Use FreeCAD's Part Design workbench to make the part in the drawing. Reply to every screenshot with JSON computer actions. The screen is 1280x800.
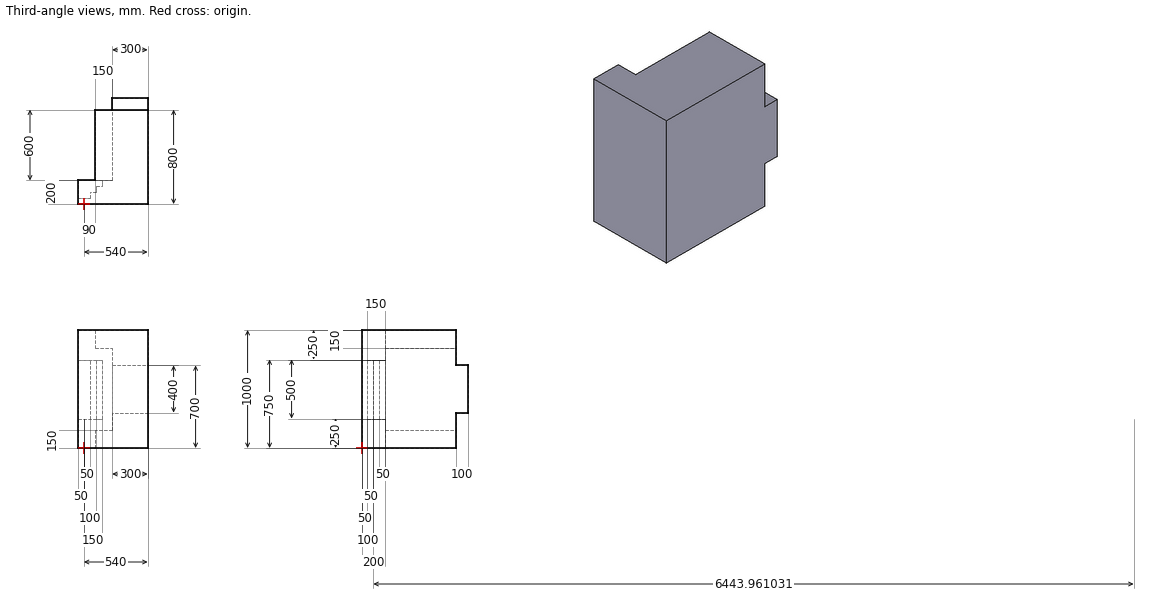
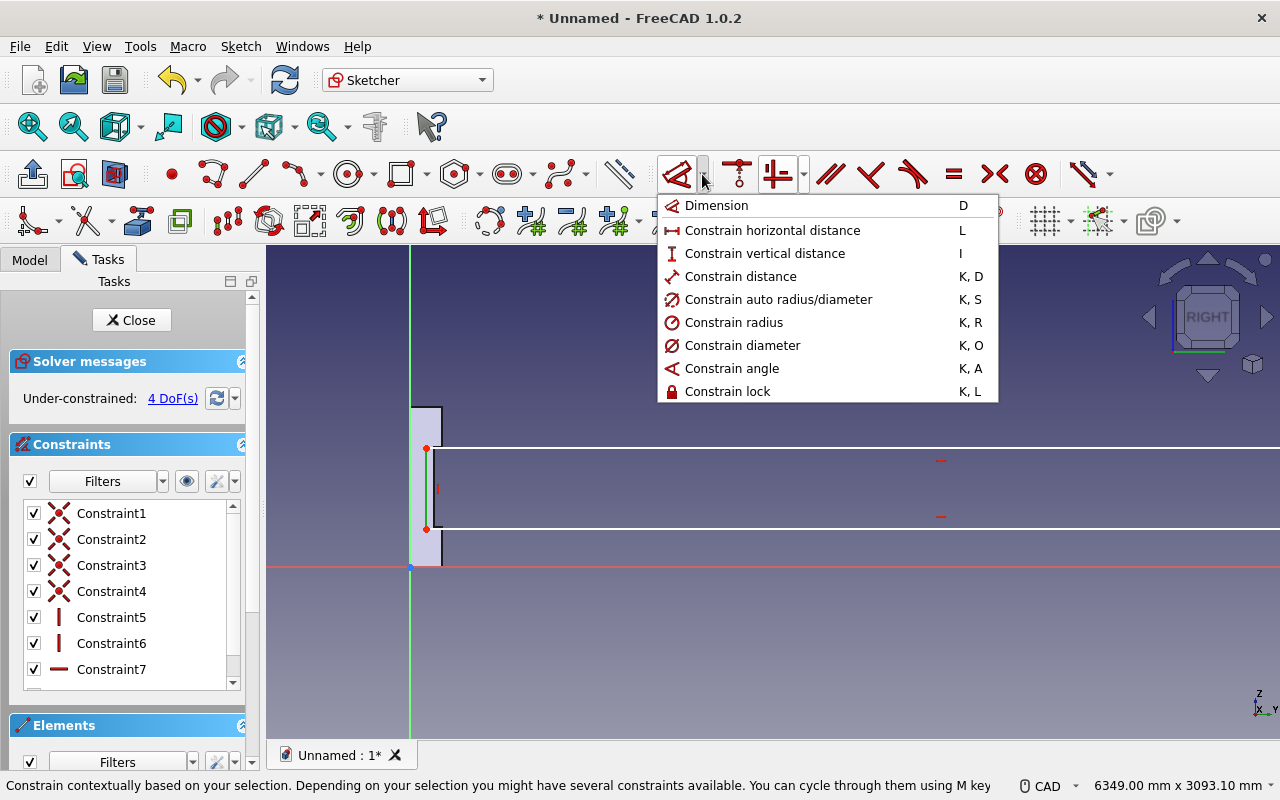
{"action": "left_click", "coordinate": [828, 254]}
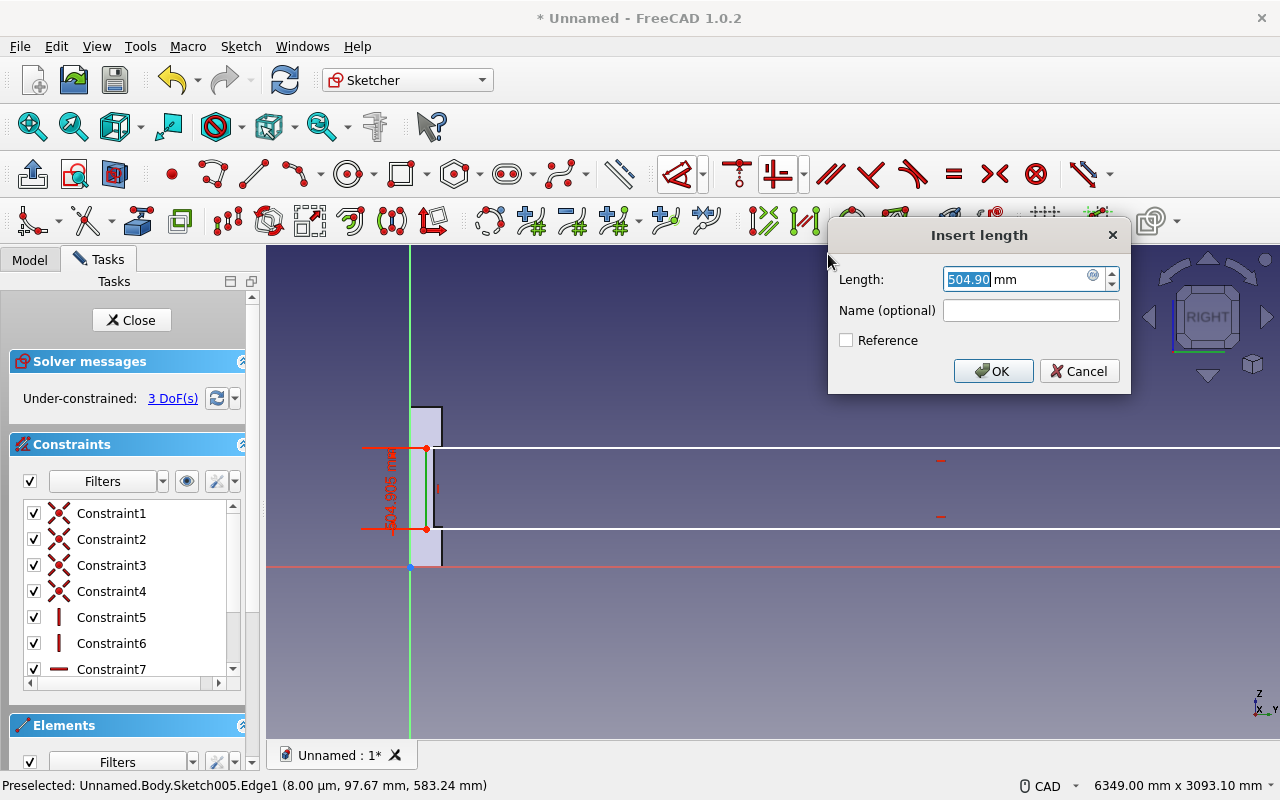
{"action": "type", "text": "500"}
{"action": "key", "text": "Return"}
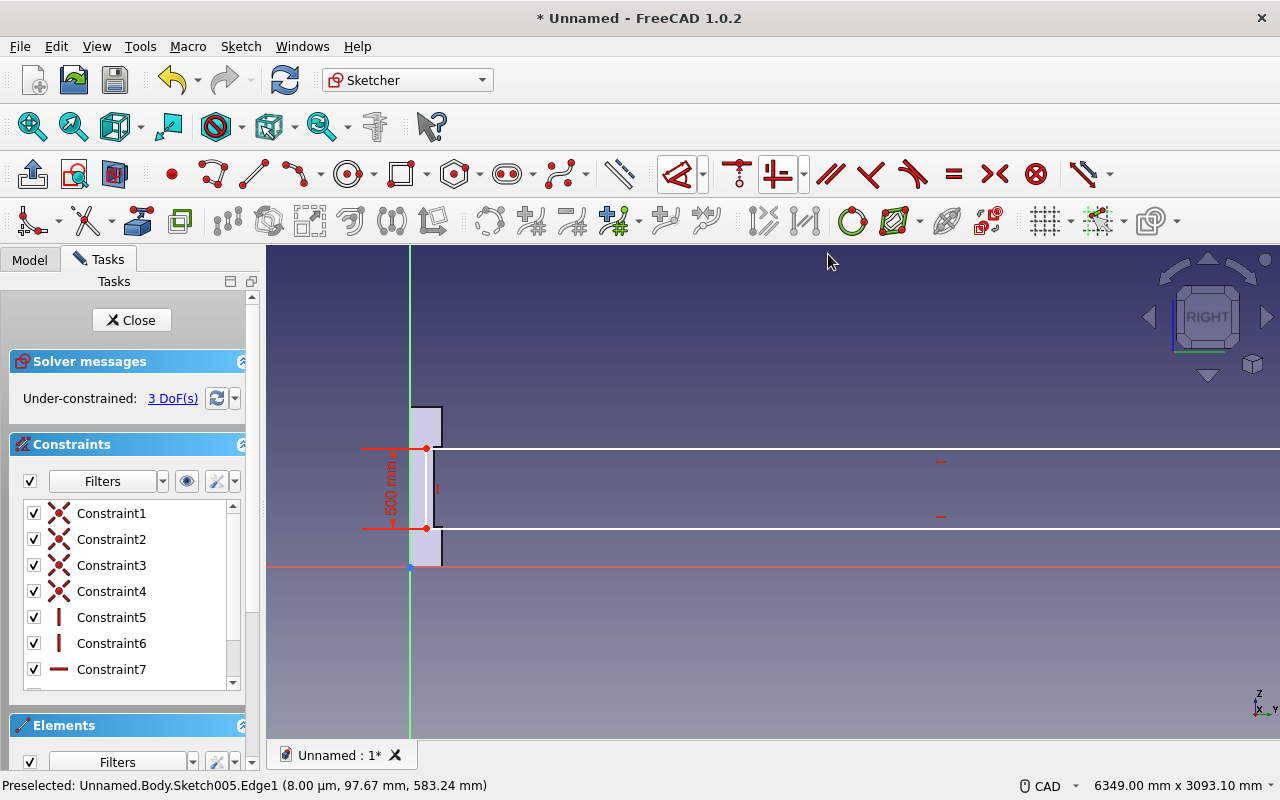
{"action": "scroll", "coordinate": [426, 449], "scroll_direction": "up", "scroll_amount": 5}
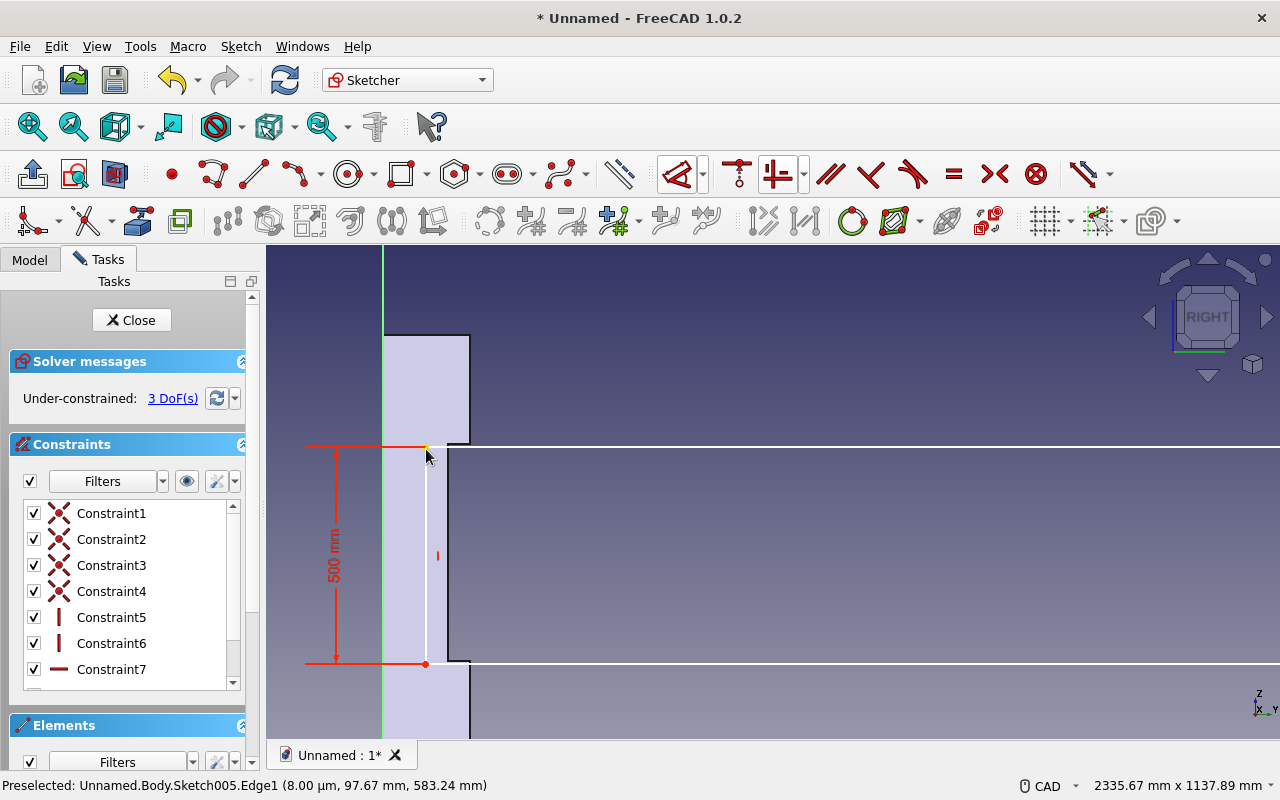
{"action": "left_click", "coordinate": [426, 447]}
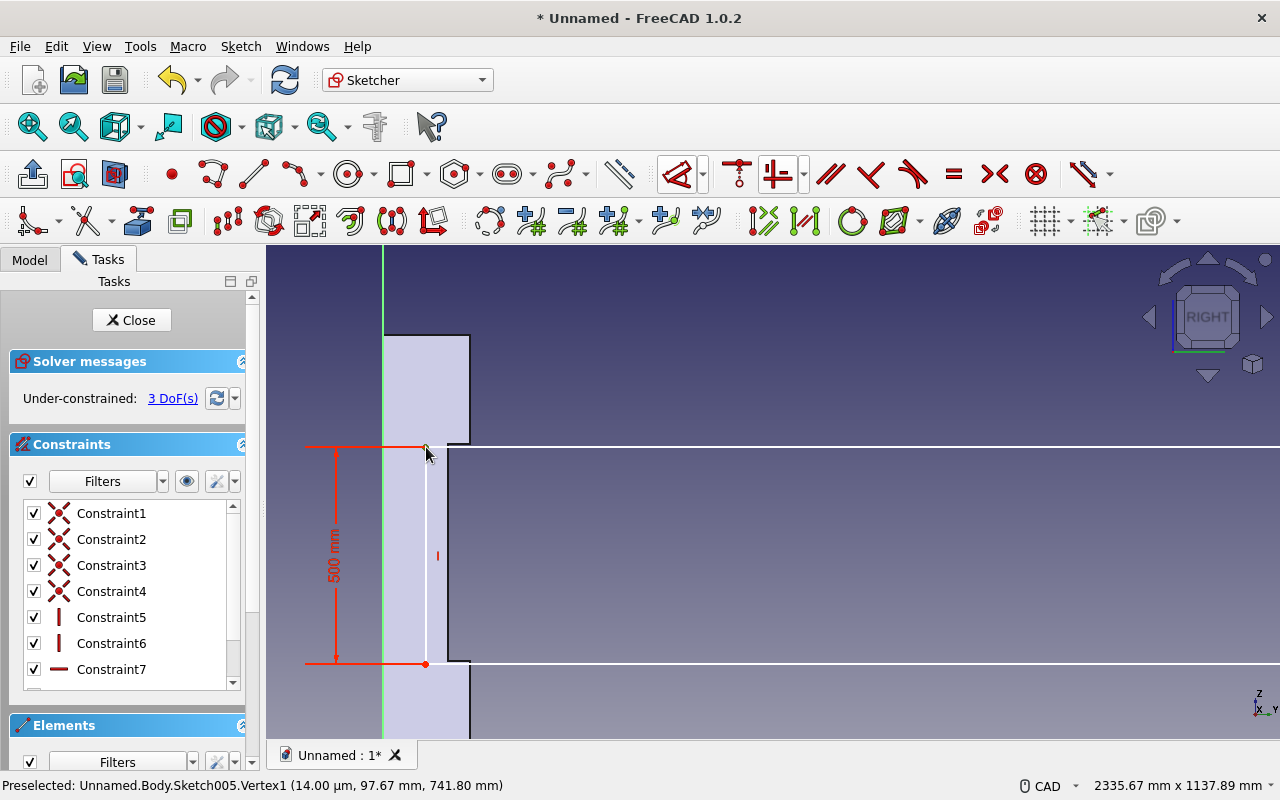
{"action": "left_click", "coordinate": [702, 174]}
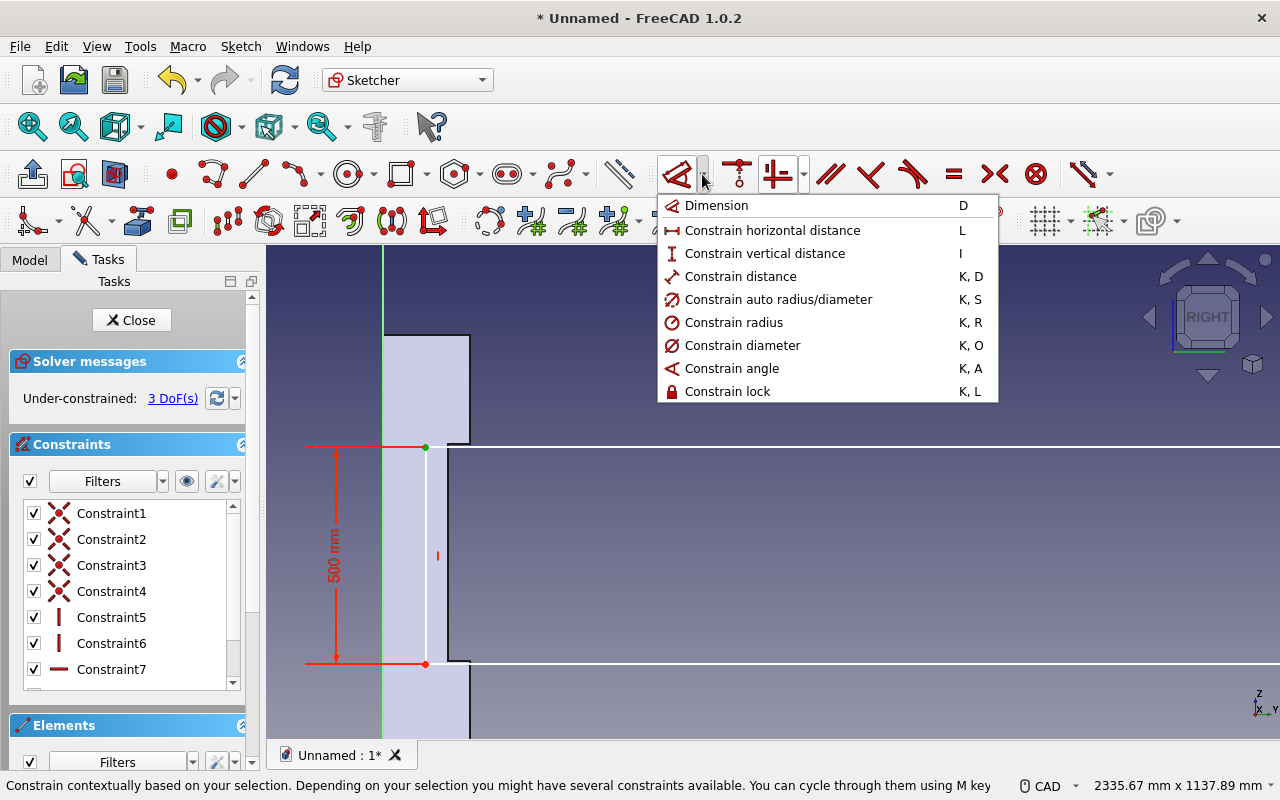
{"action": "left_click", "coordinate": [828, 230]}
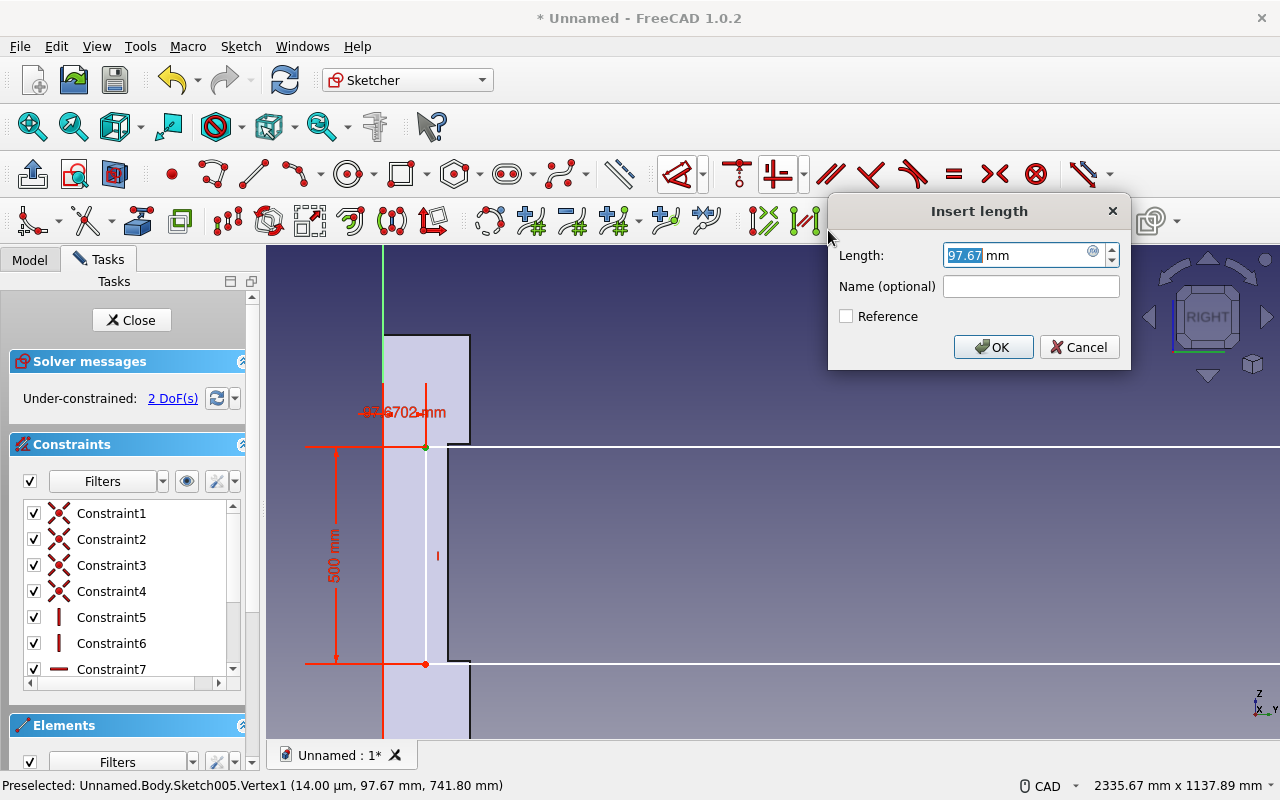
{"action": "type", "text": "100"}
{"action": "key", "text": "Return"}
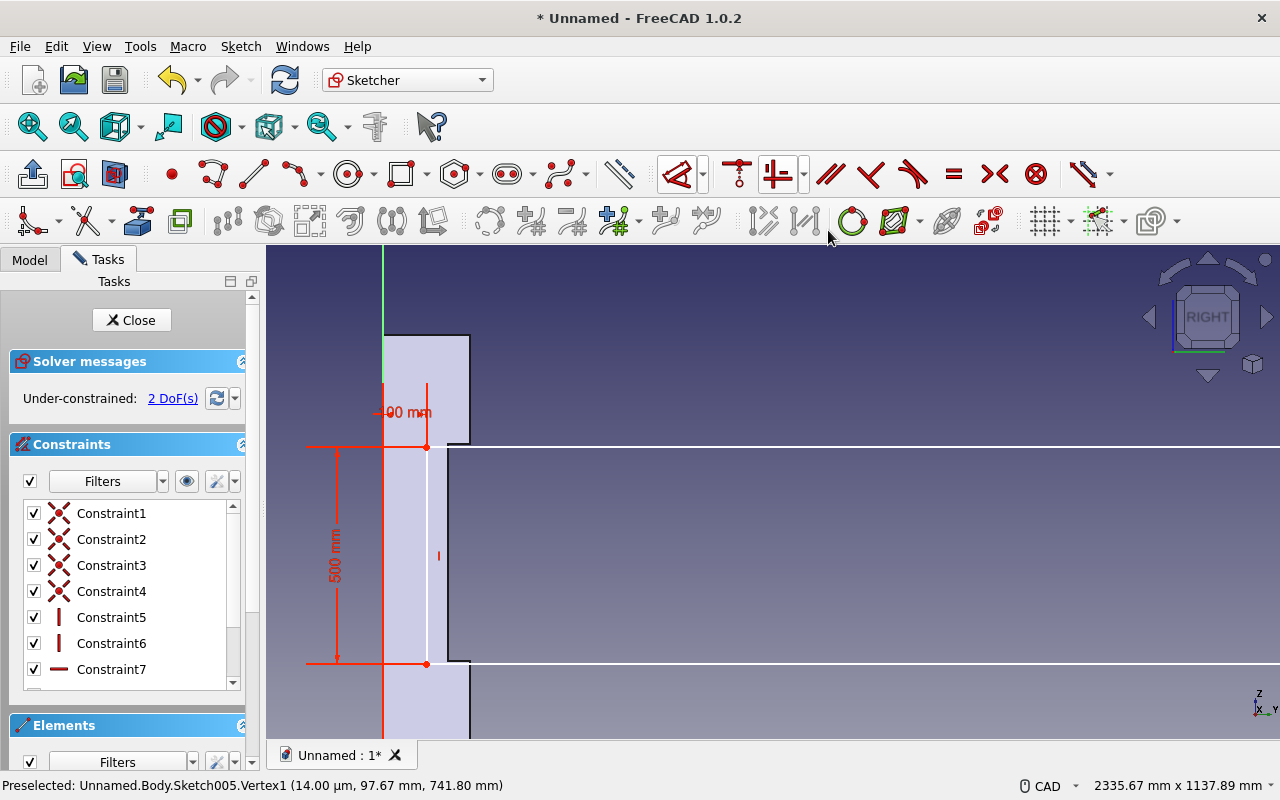
{"action": "scroll", "coordinate": [426, 463], "scroll_direction": "down", "scroll_amount": 8}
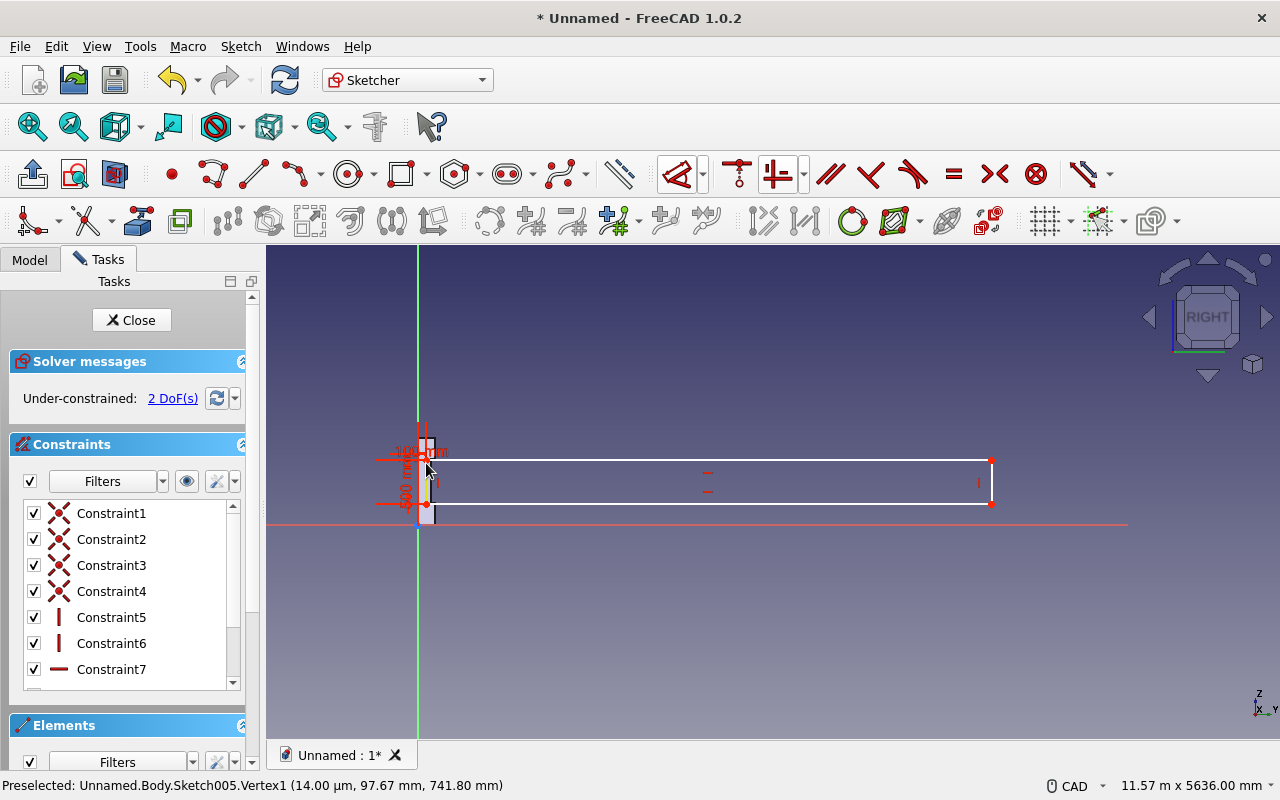
{"action": "left_click", "coordinate": [426, 460]}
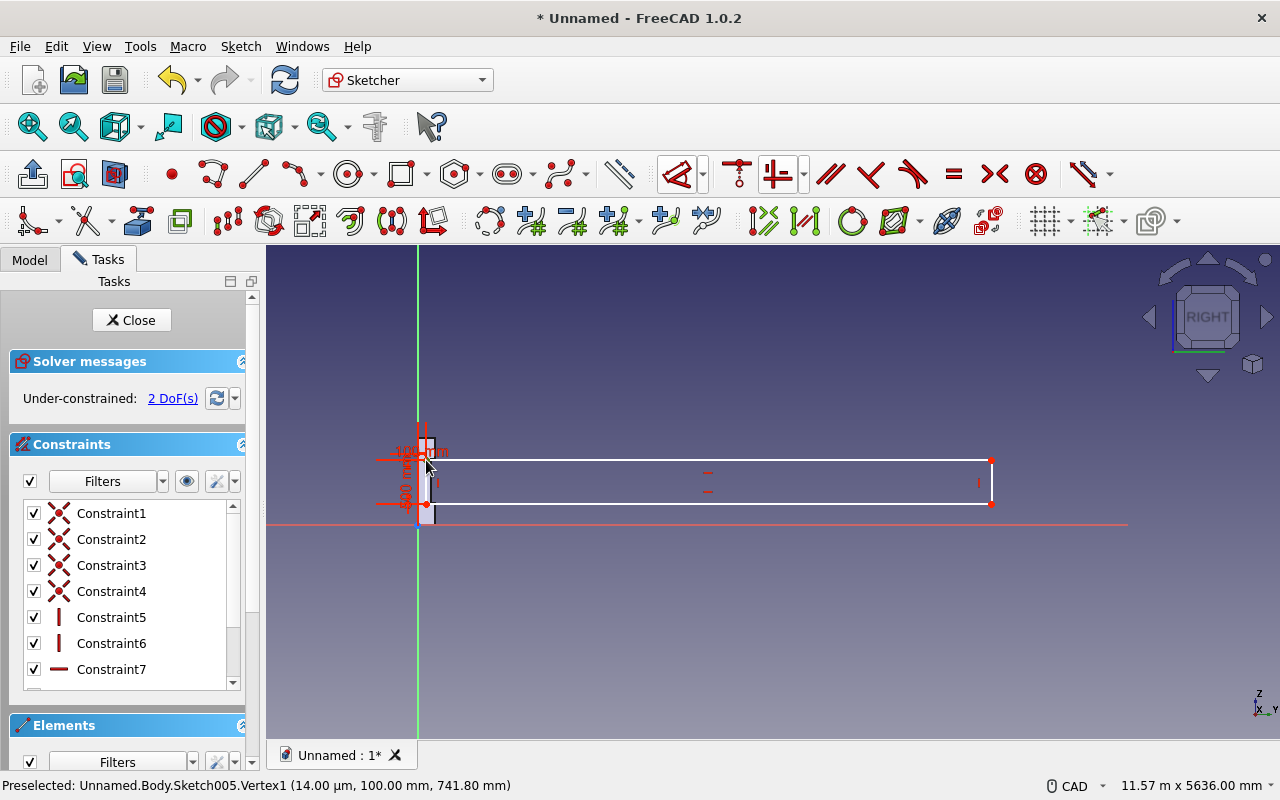
{"action": "left_click", "coordinate": [702, 174]}